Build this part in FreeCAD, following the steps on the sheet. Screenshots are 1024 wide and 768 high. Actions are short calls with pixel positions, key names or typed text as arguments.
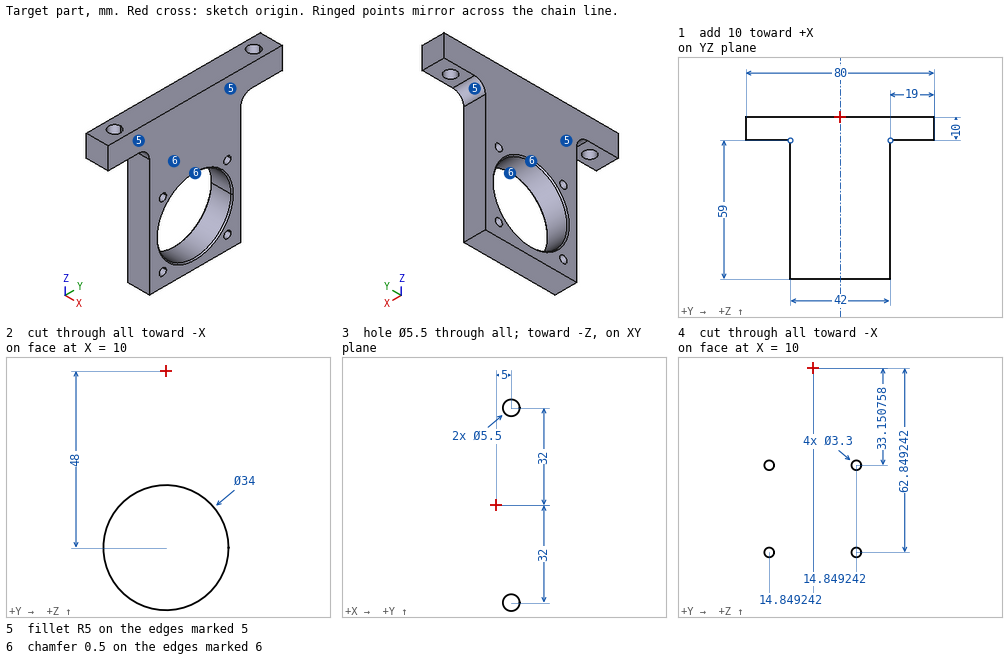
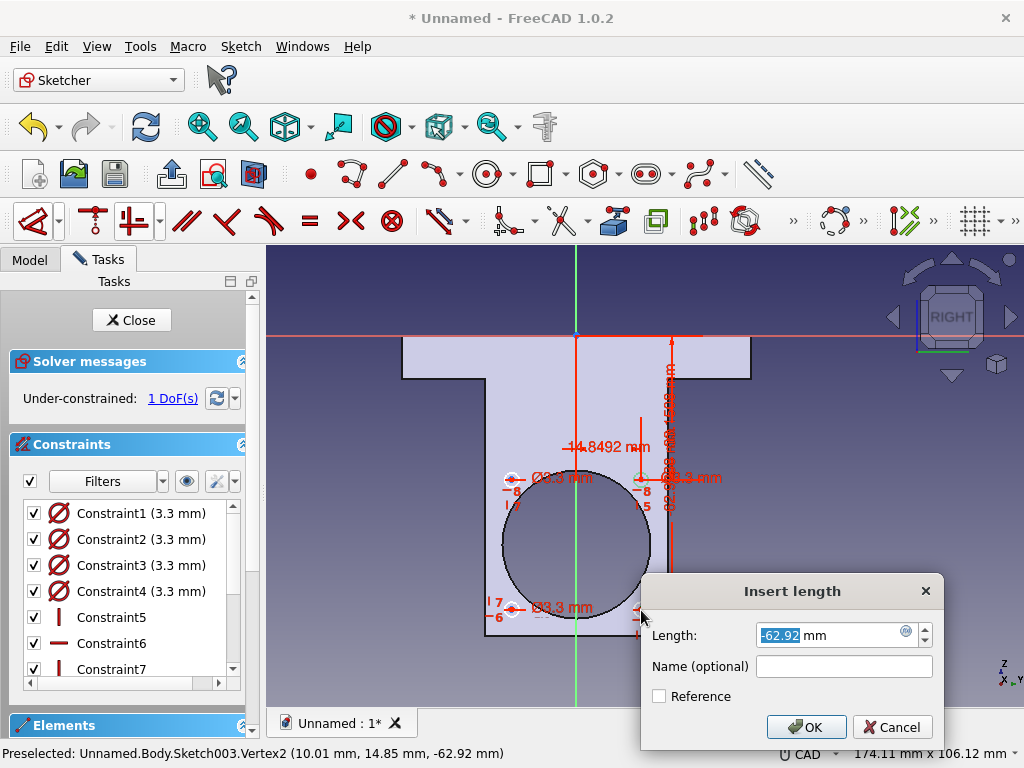
text(-62.849242)
key(Return)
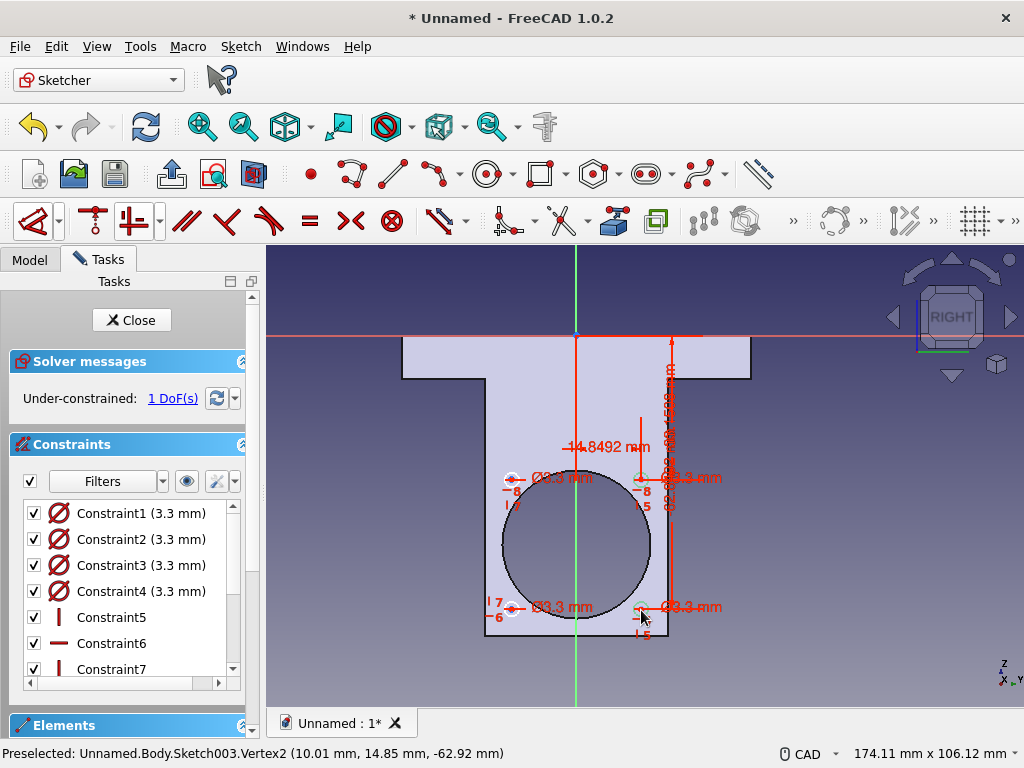
click(512, 609)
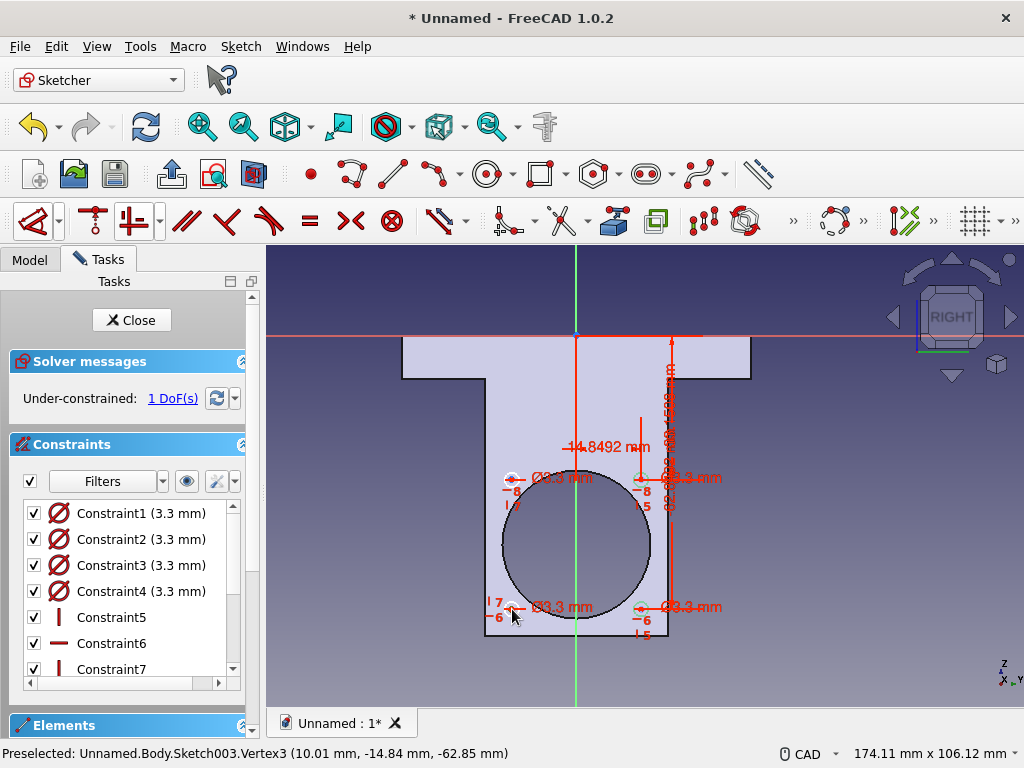
click(58, 222)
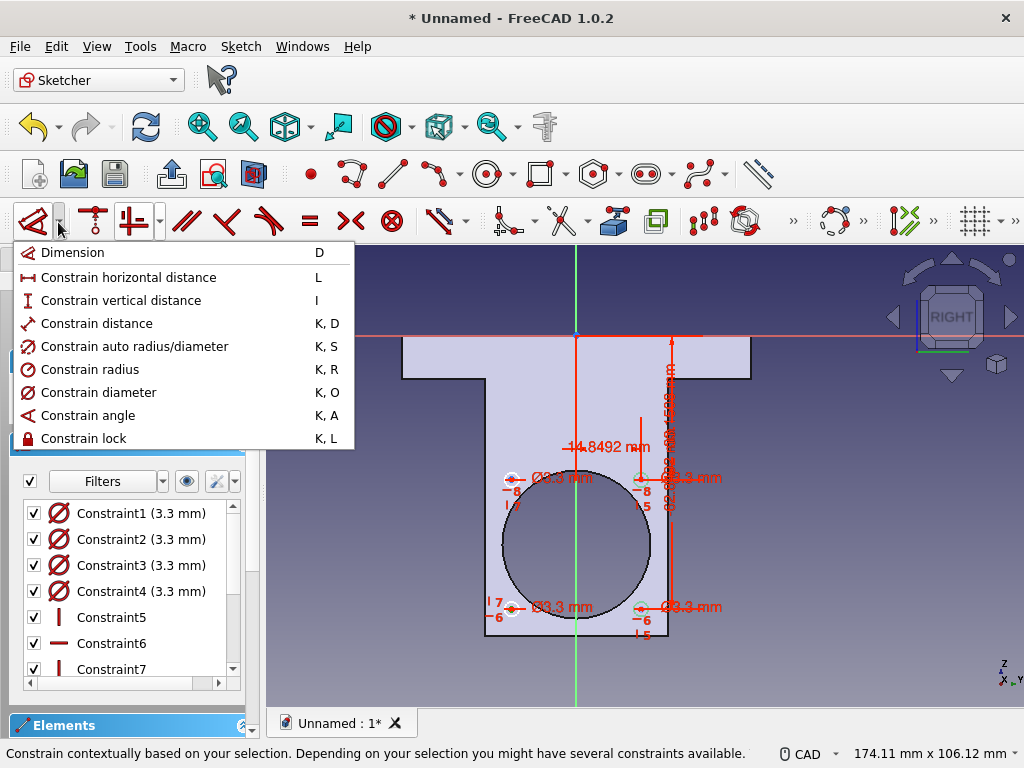
click(184, 278)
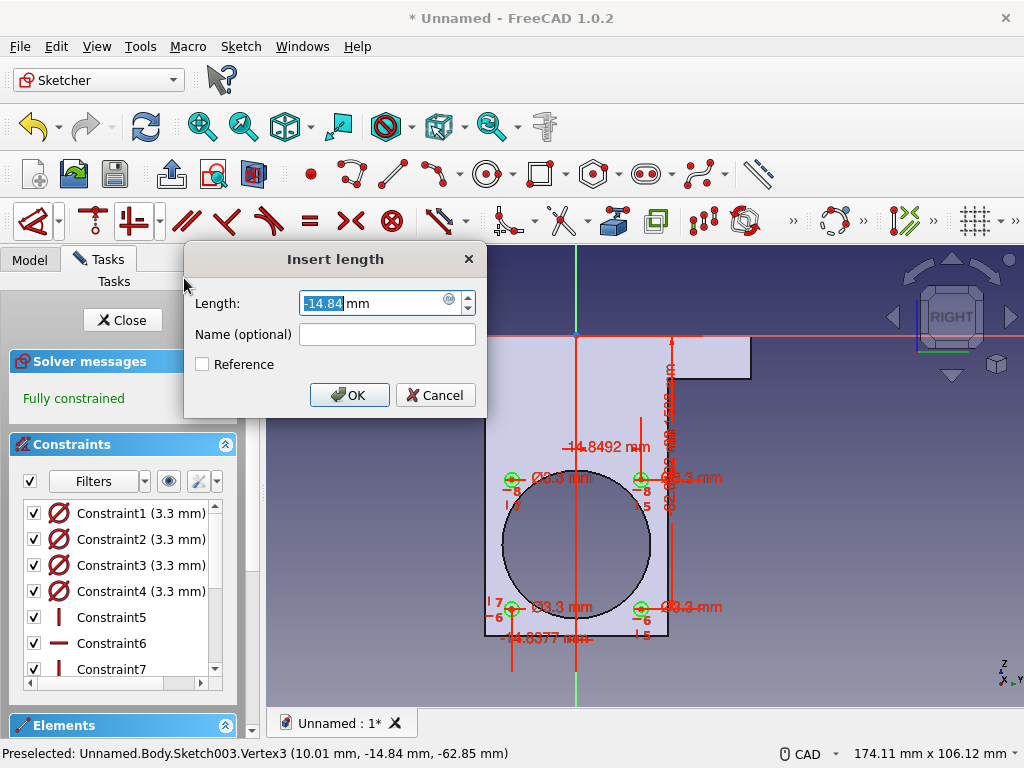
text(-14.849242)
key(Return)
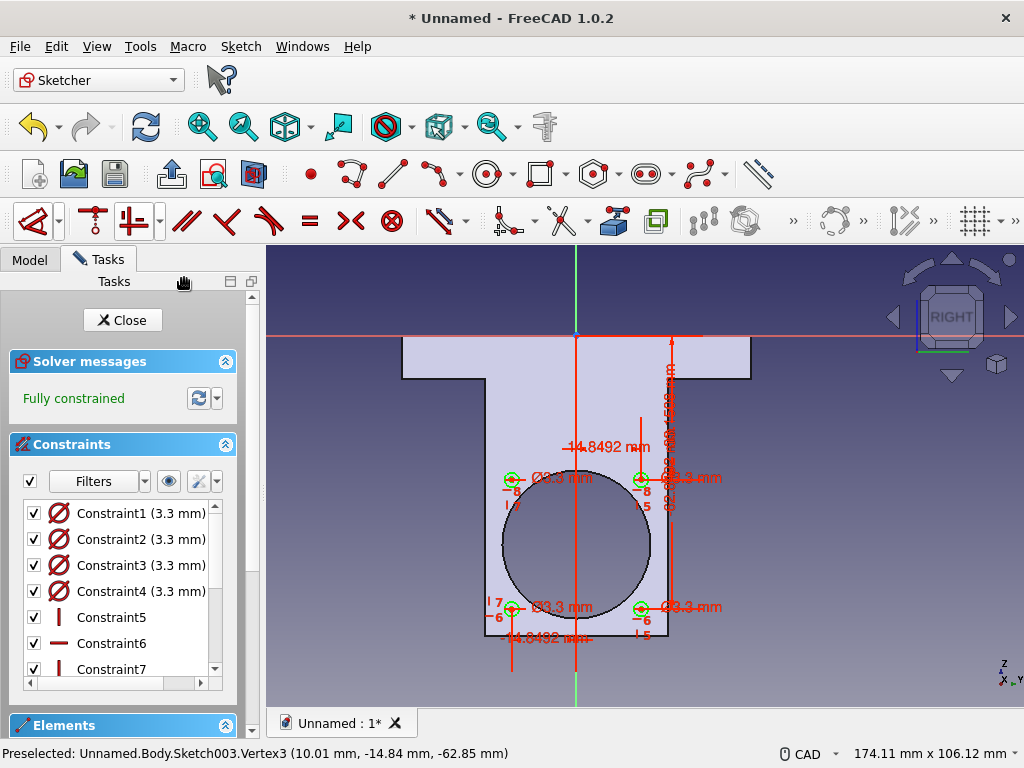
click(123, 320)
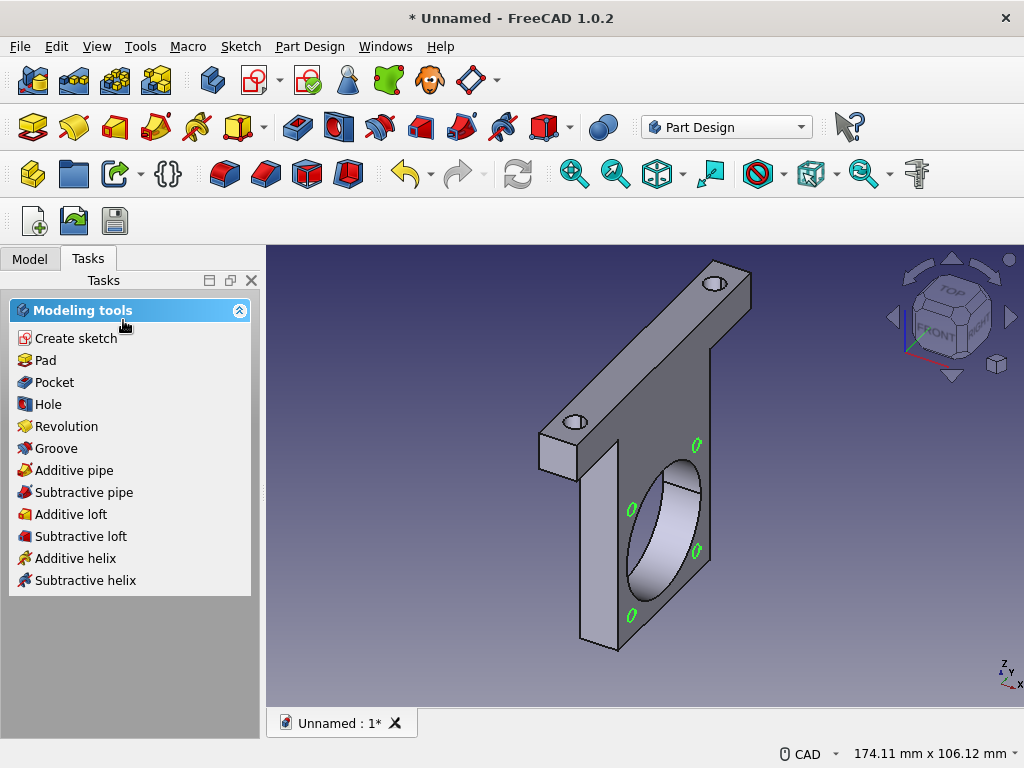
click(298, 128)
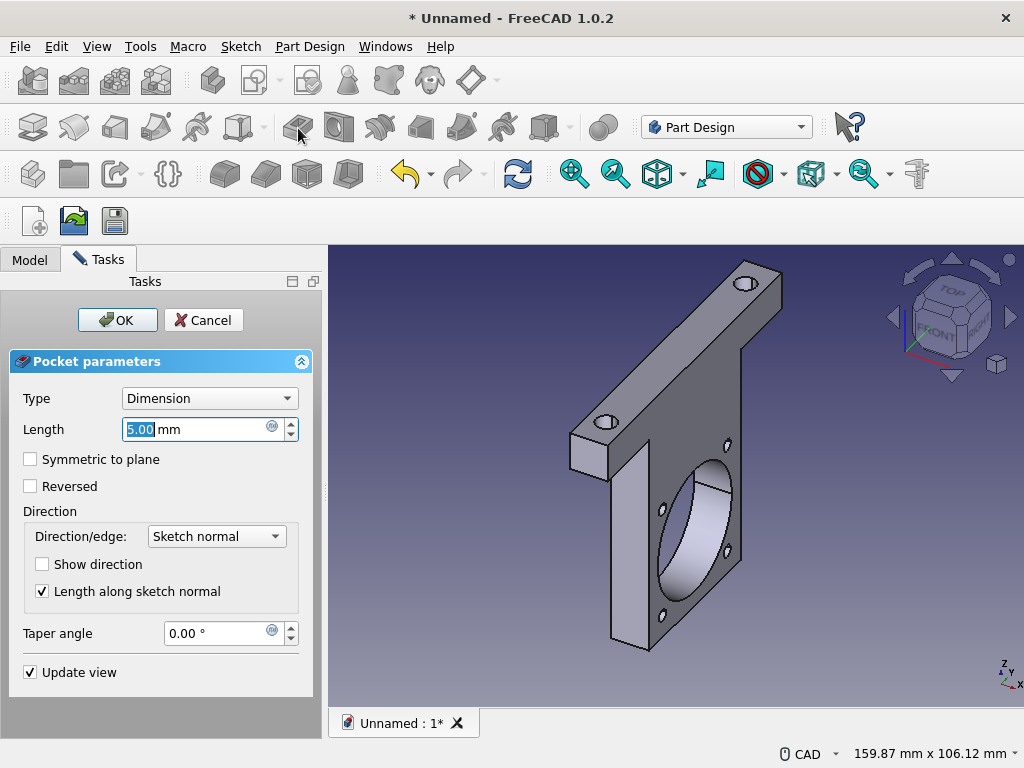
click(210, 398)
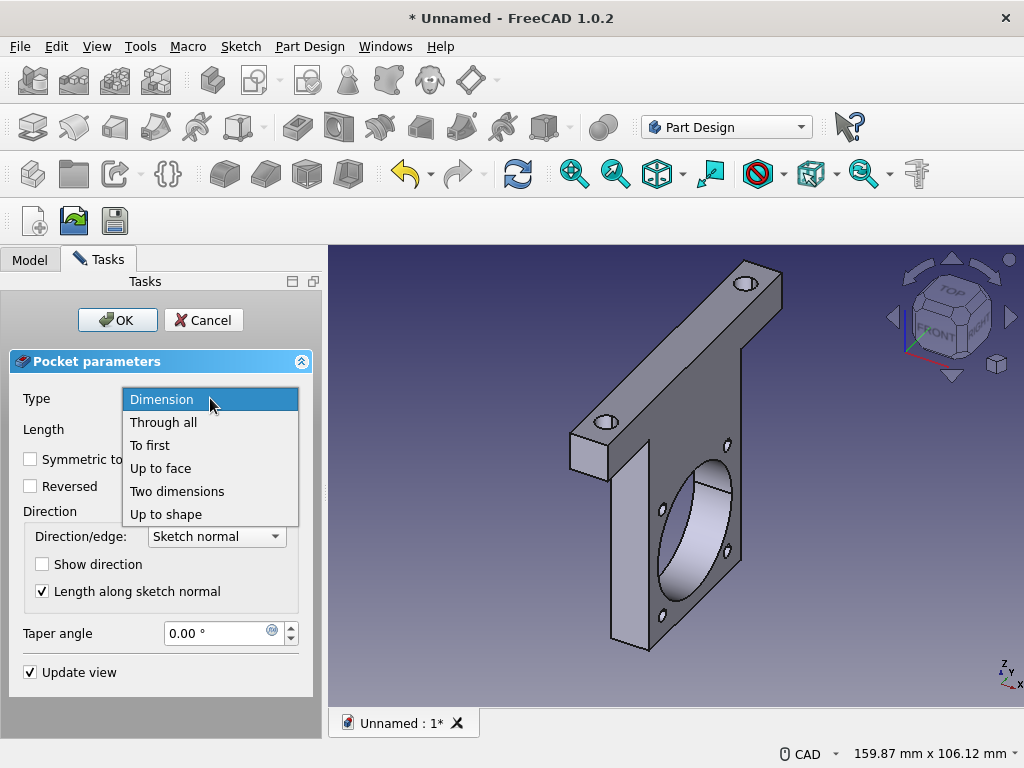
click(208, 422)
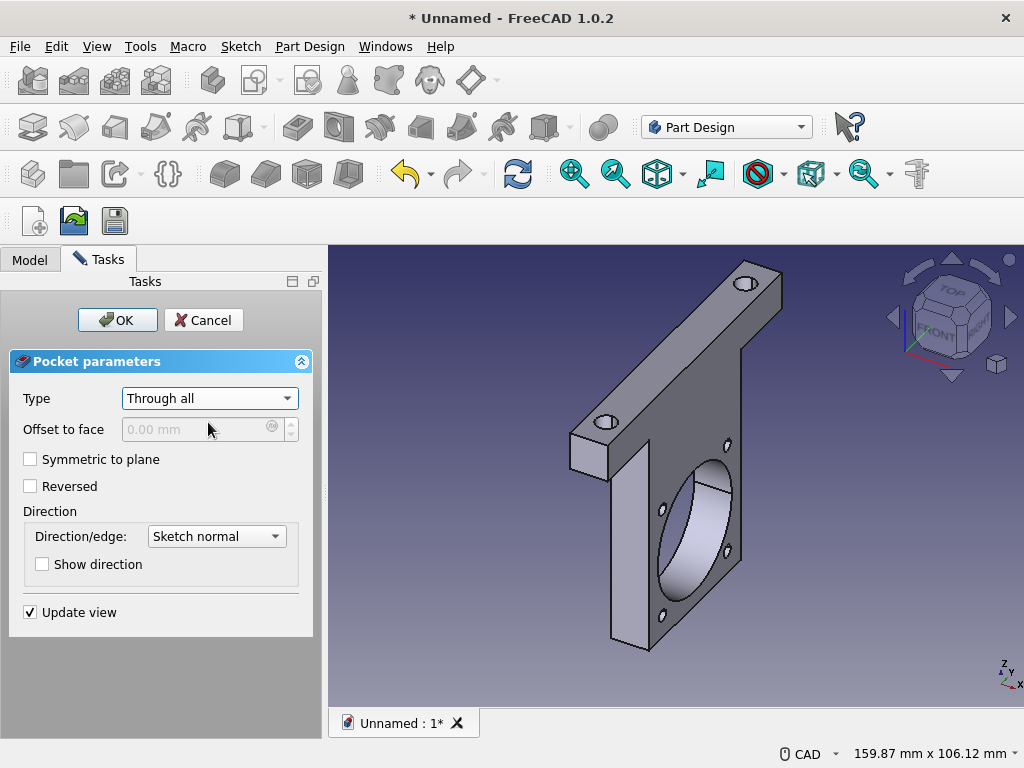
click(118, 320)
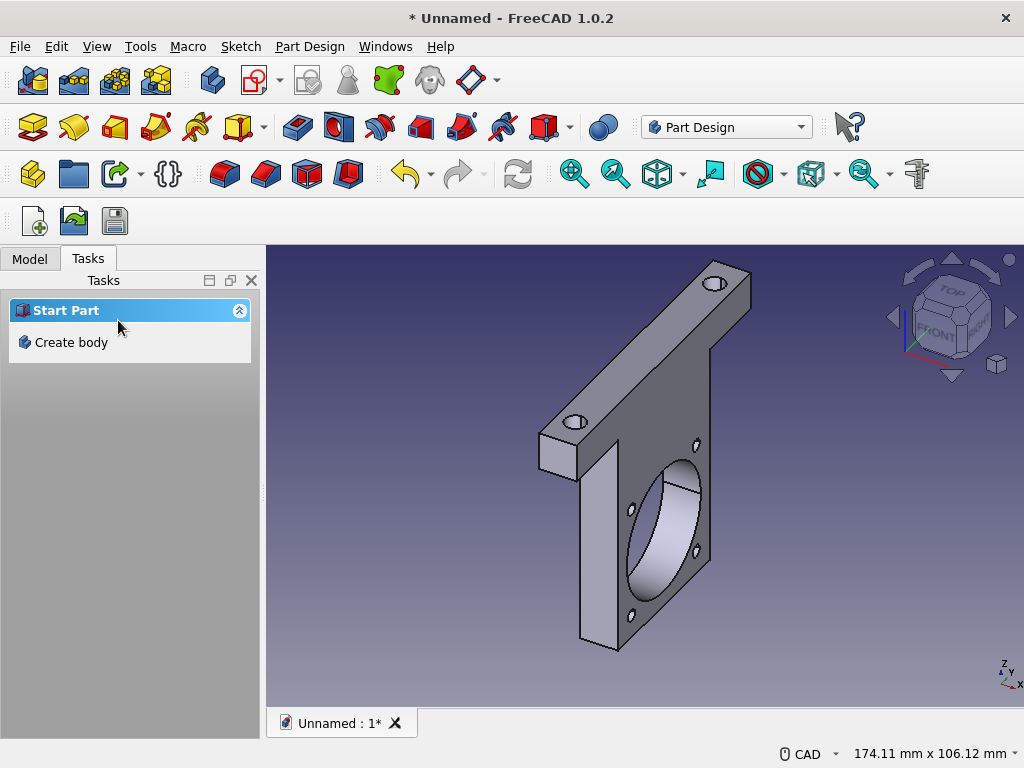
key(0)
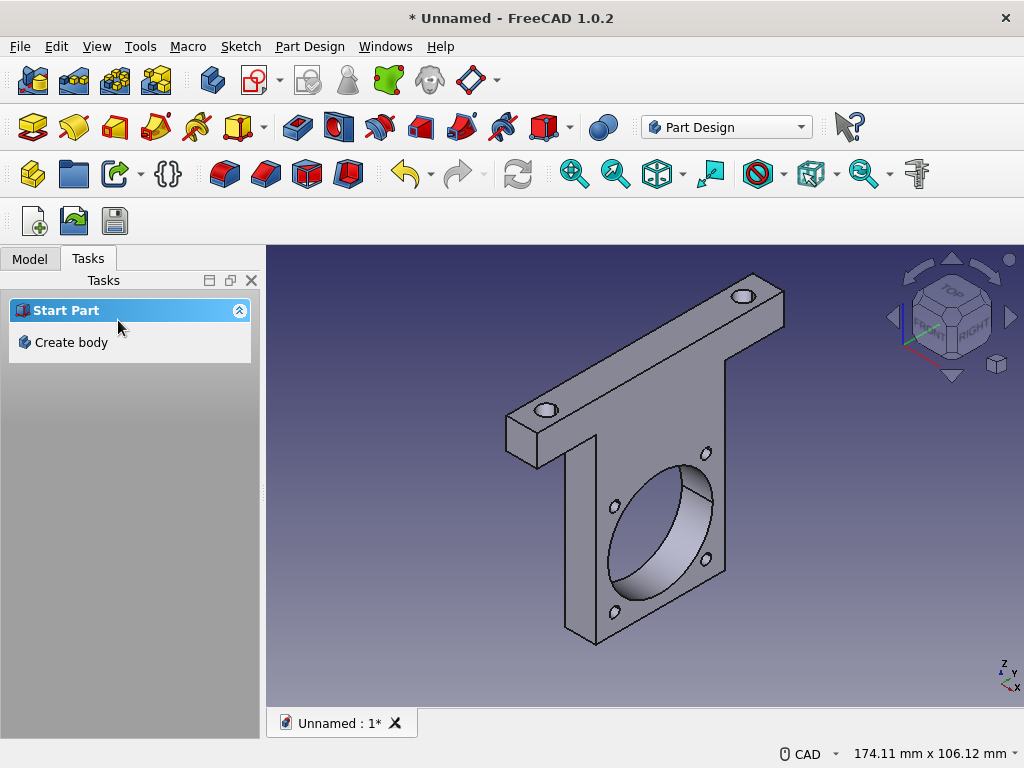
key(2)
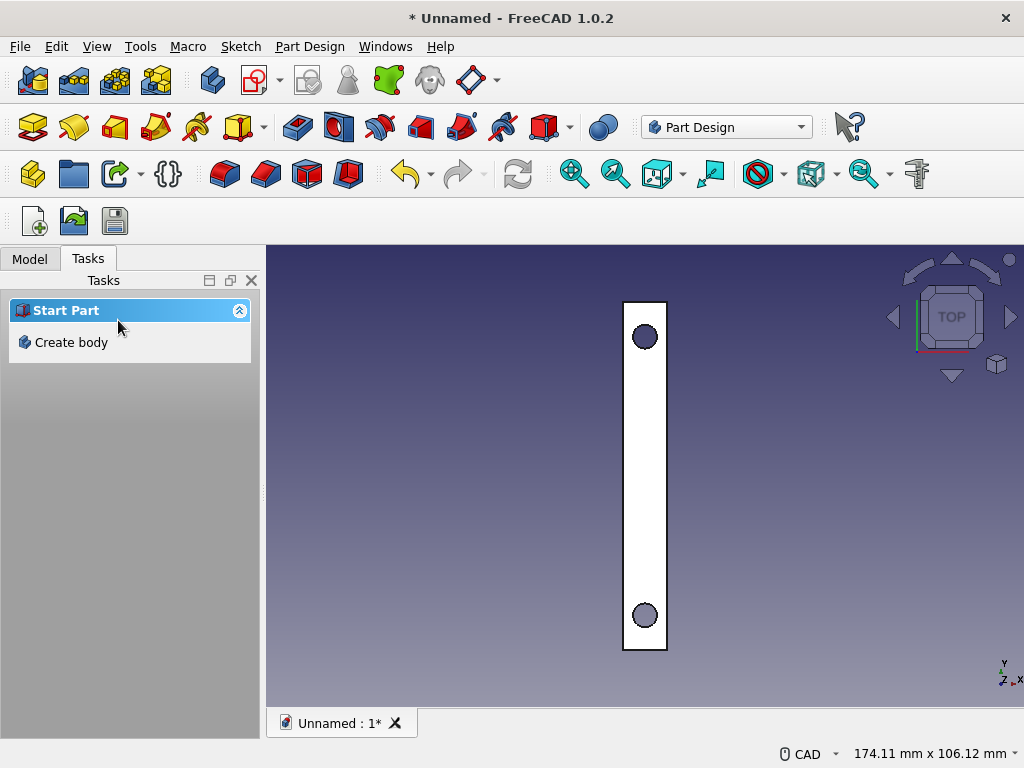
key(1)